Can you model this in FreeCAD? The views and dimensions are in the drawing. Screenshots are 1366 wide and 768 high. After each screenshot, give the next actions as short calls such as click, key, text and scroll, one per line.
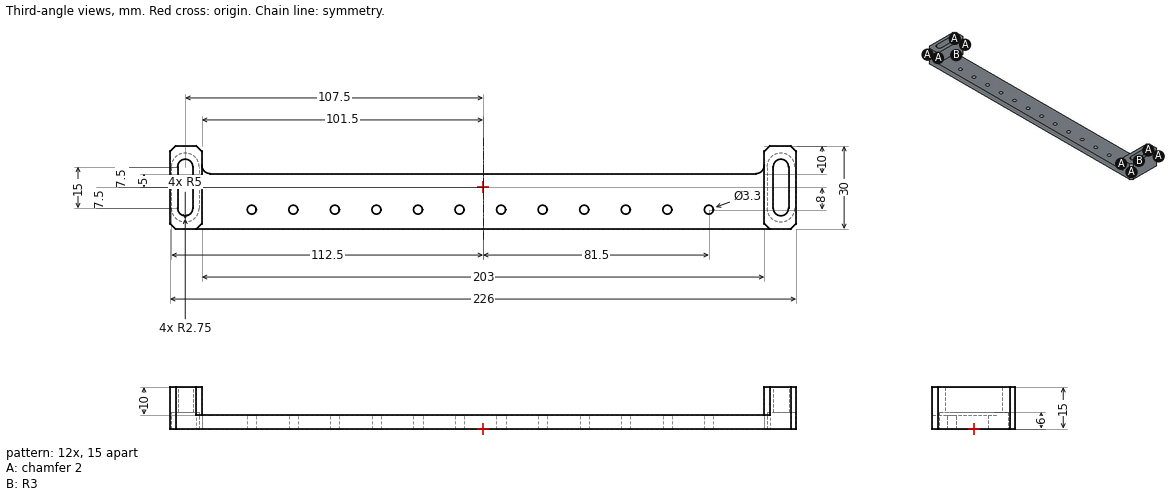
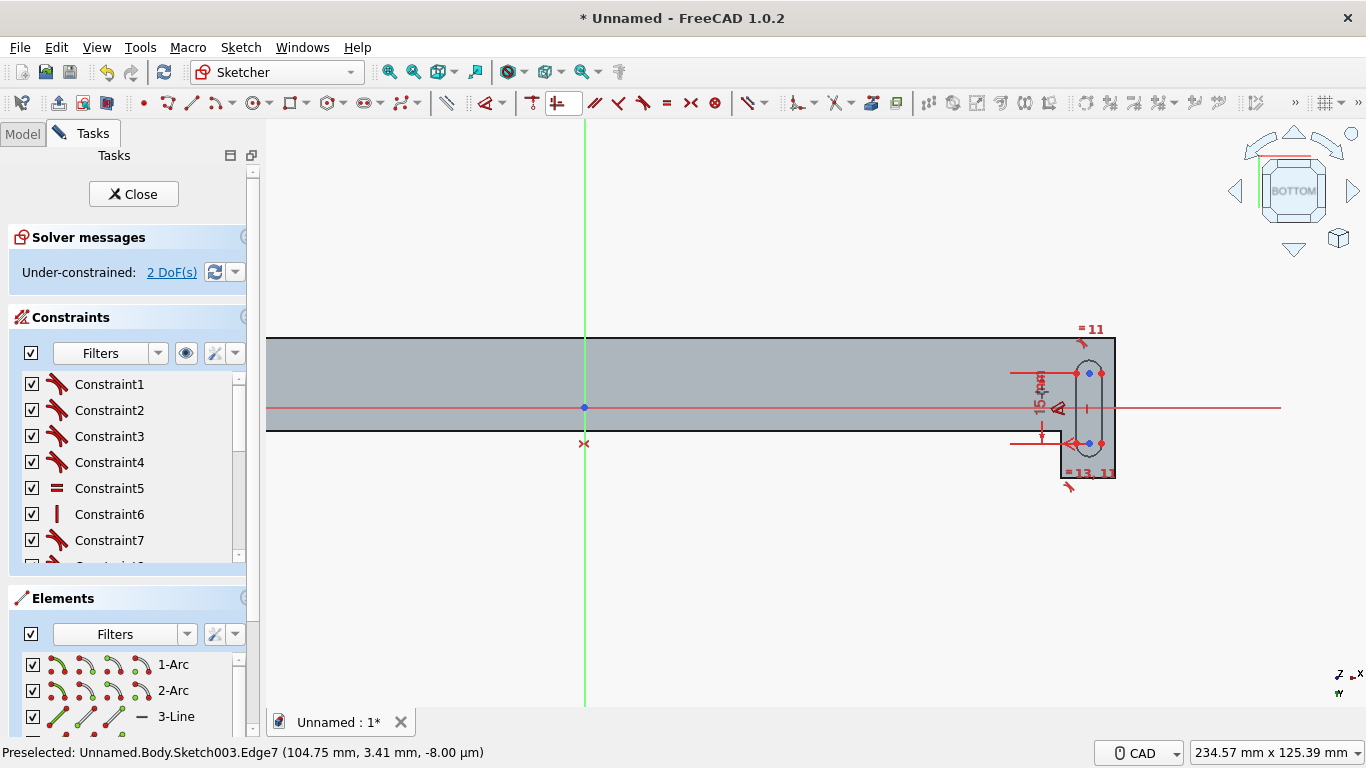
scroll(1078, 423, down, 2)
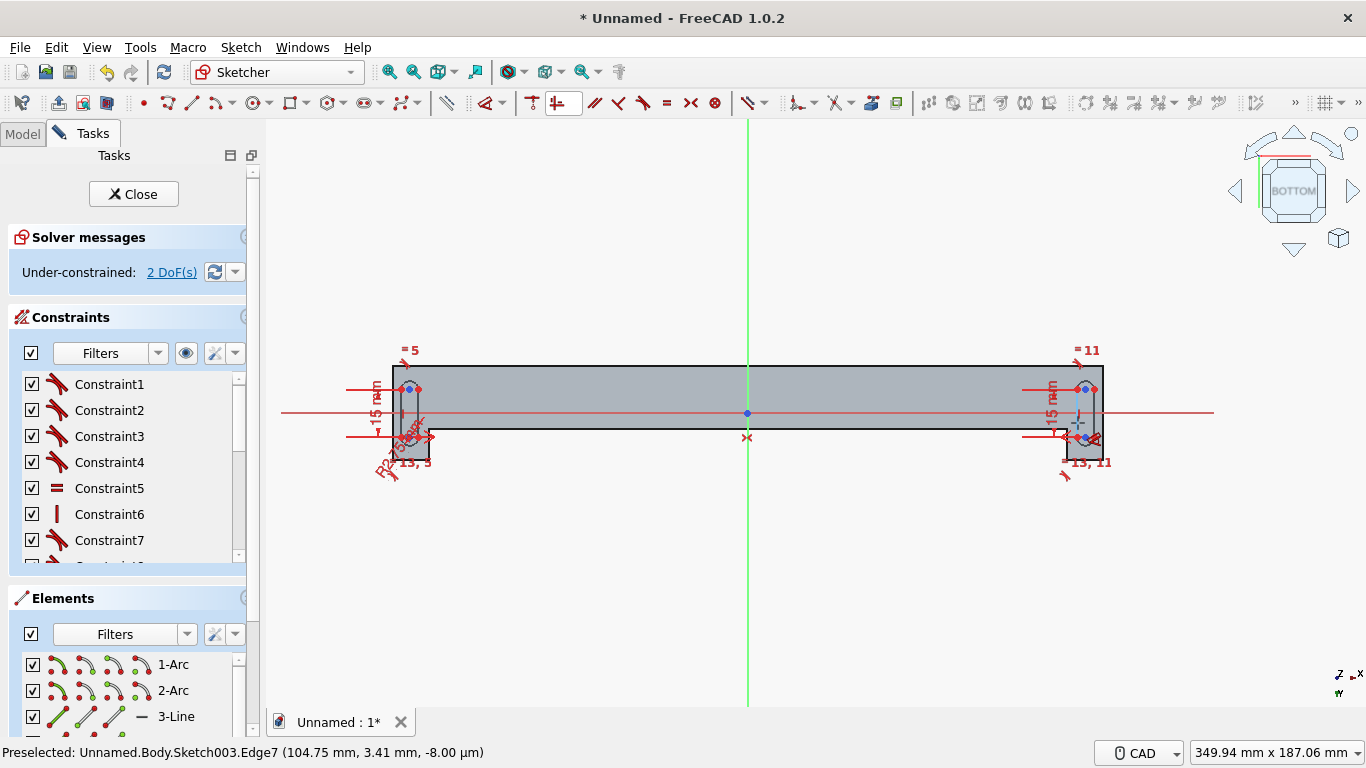
scroll(401, 437, up, 3)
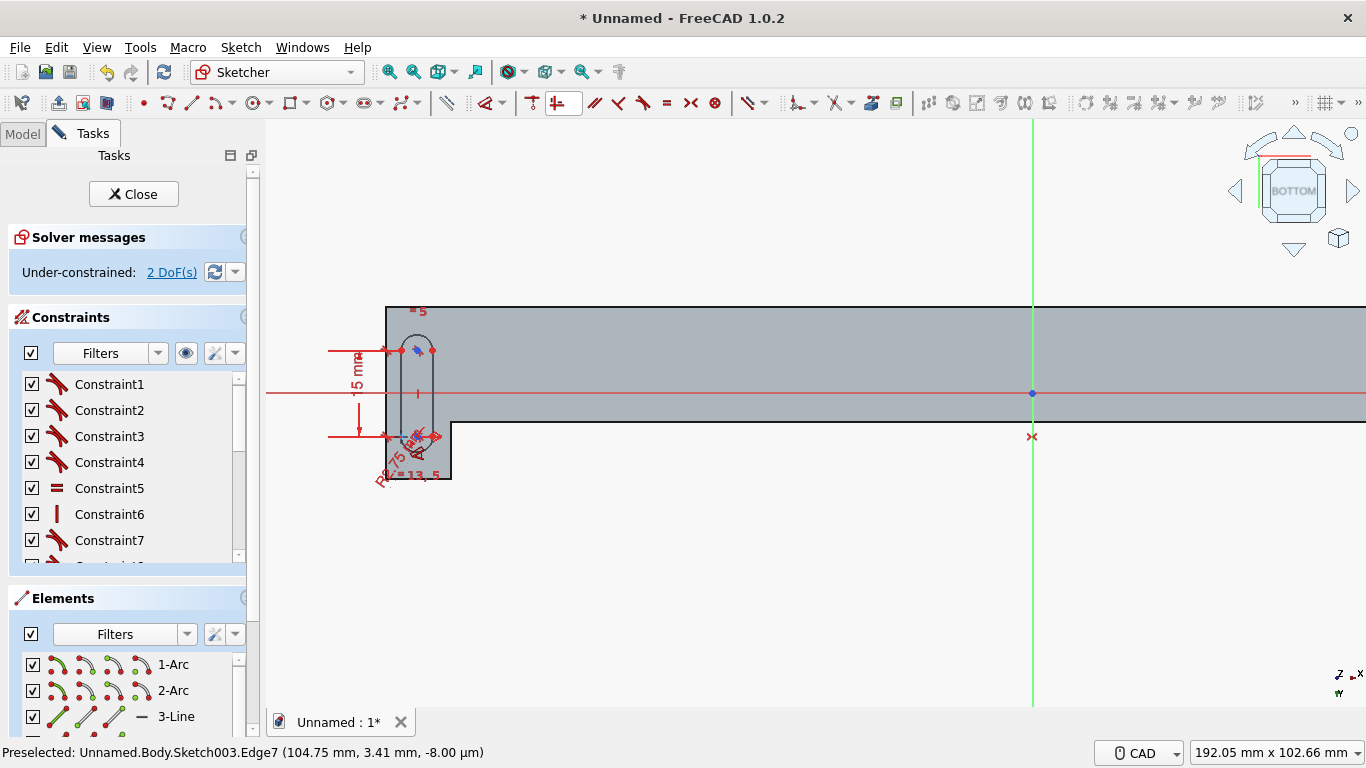
click(401, 437)
click(367, 415)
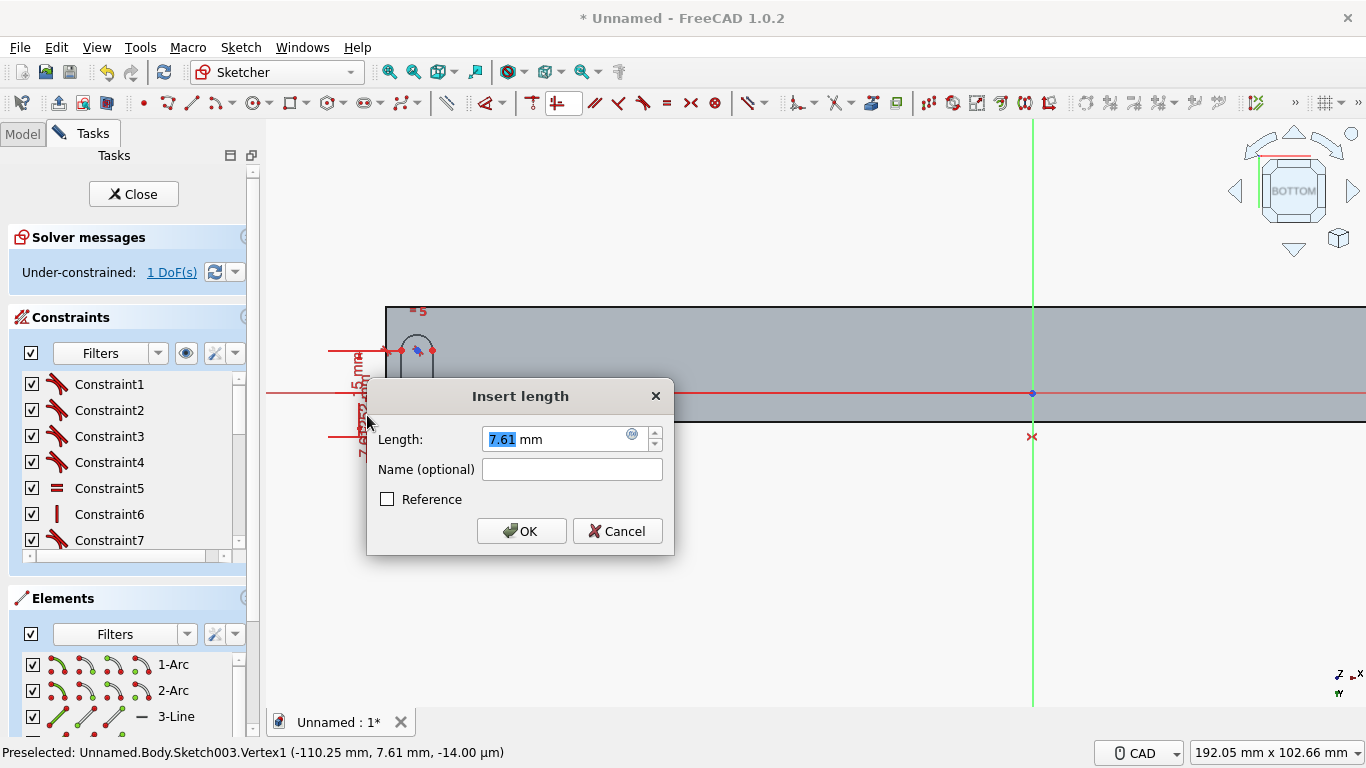
text(7.5)
key(Return)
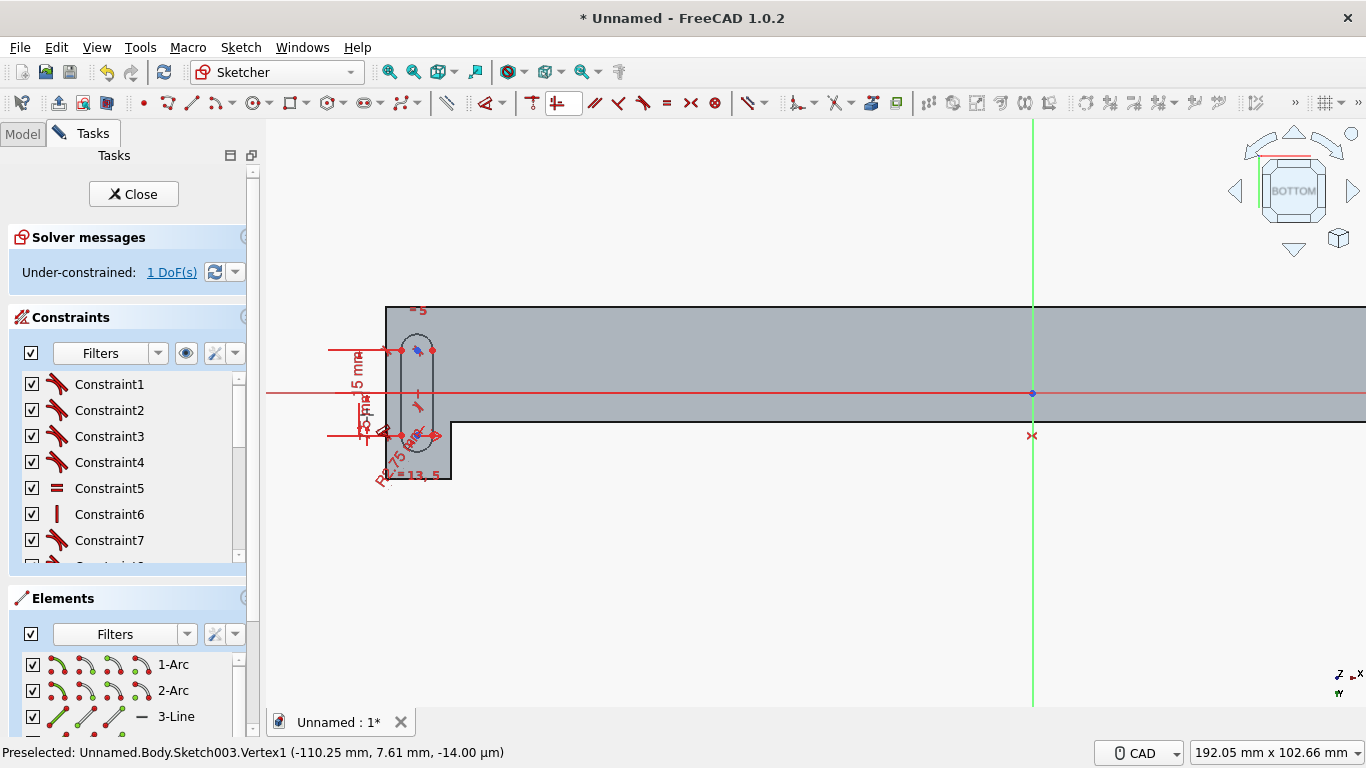
click(417, 436)
click(725, 470)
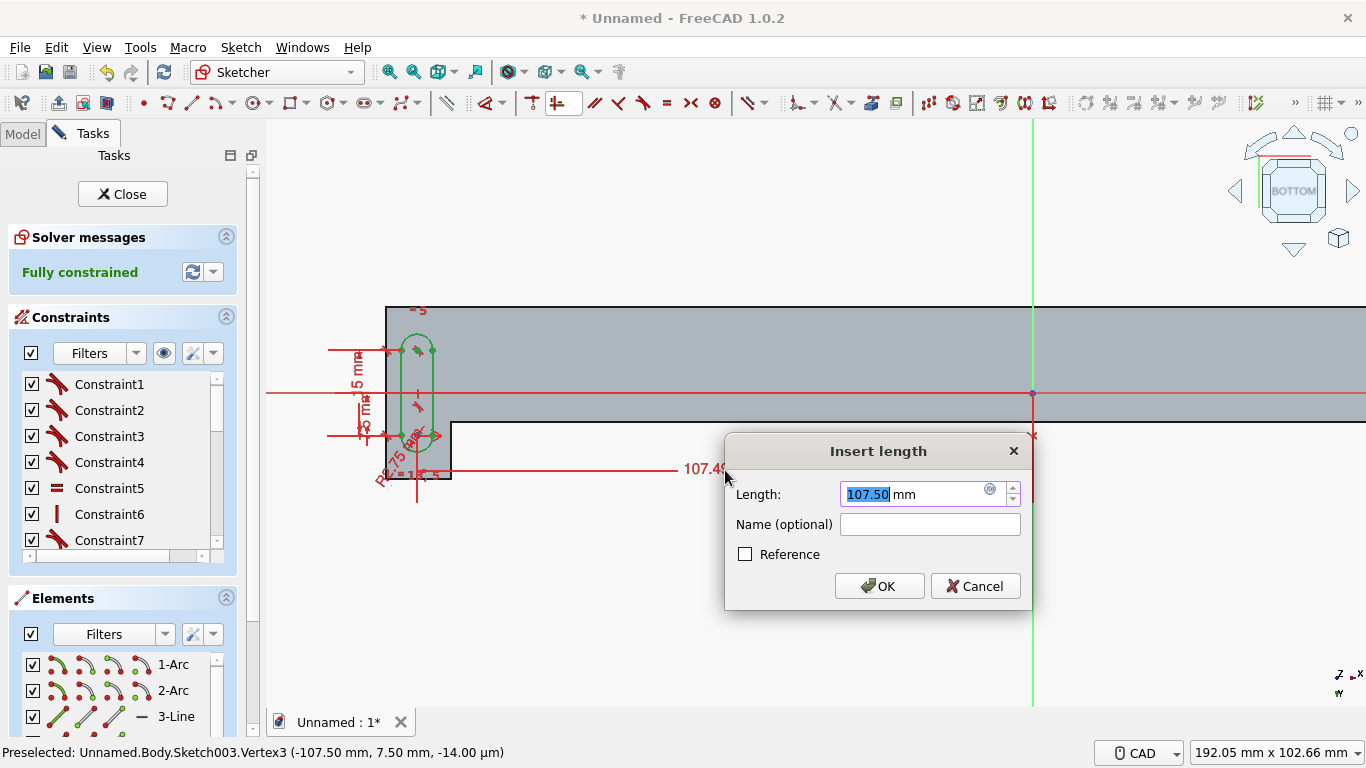
text(107.5)
key(Return)
key(Escape)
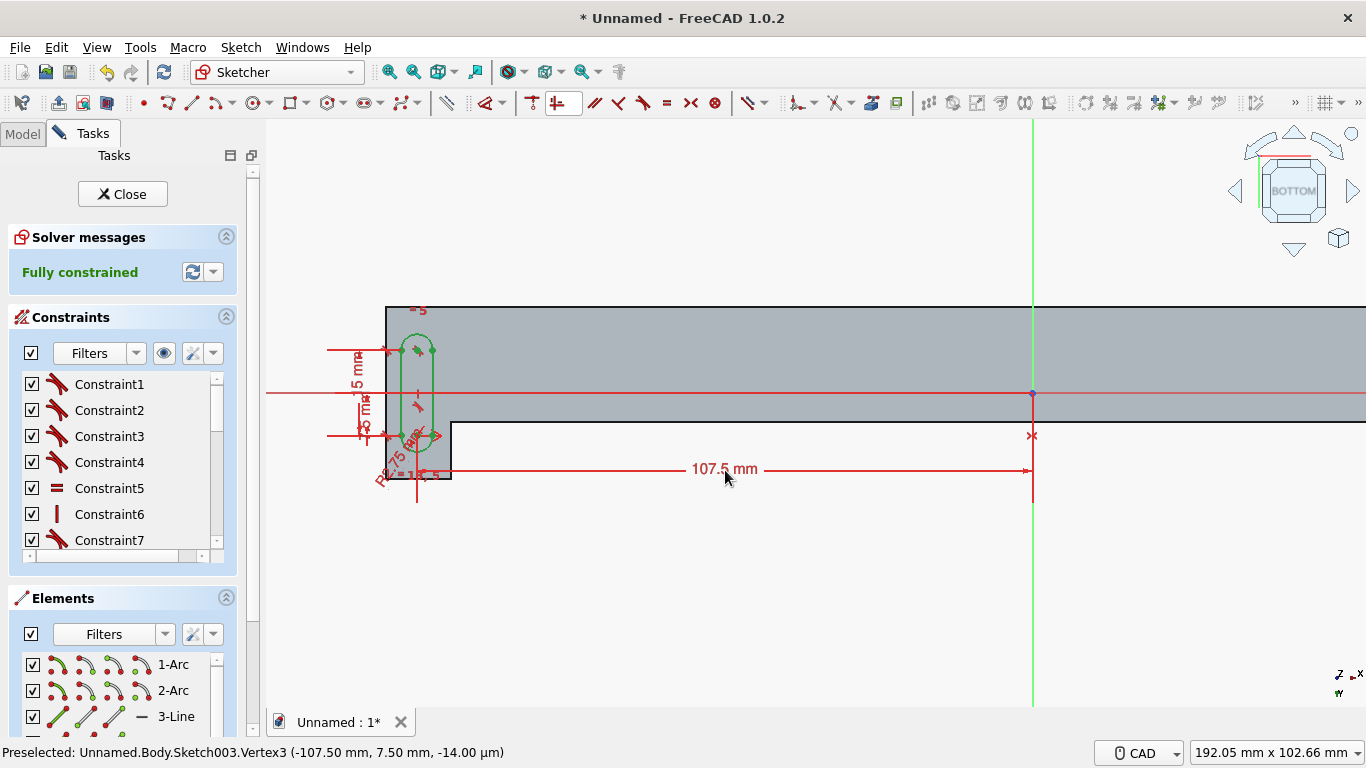
click(123, 194)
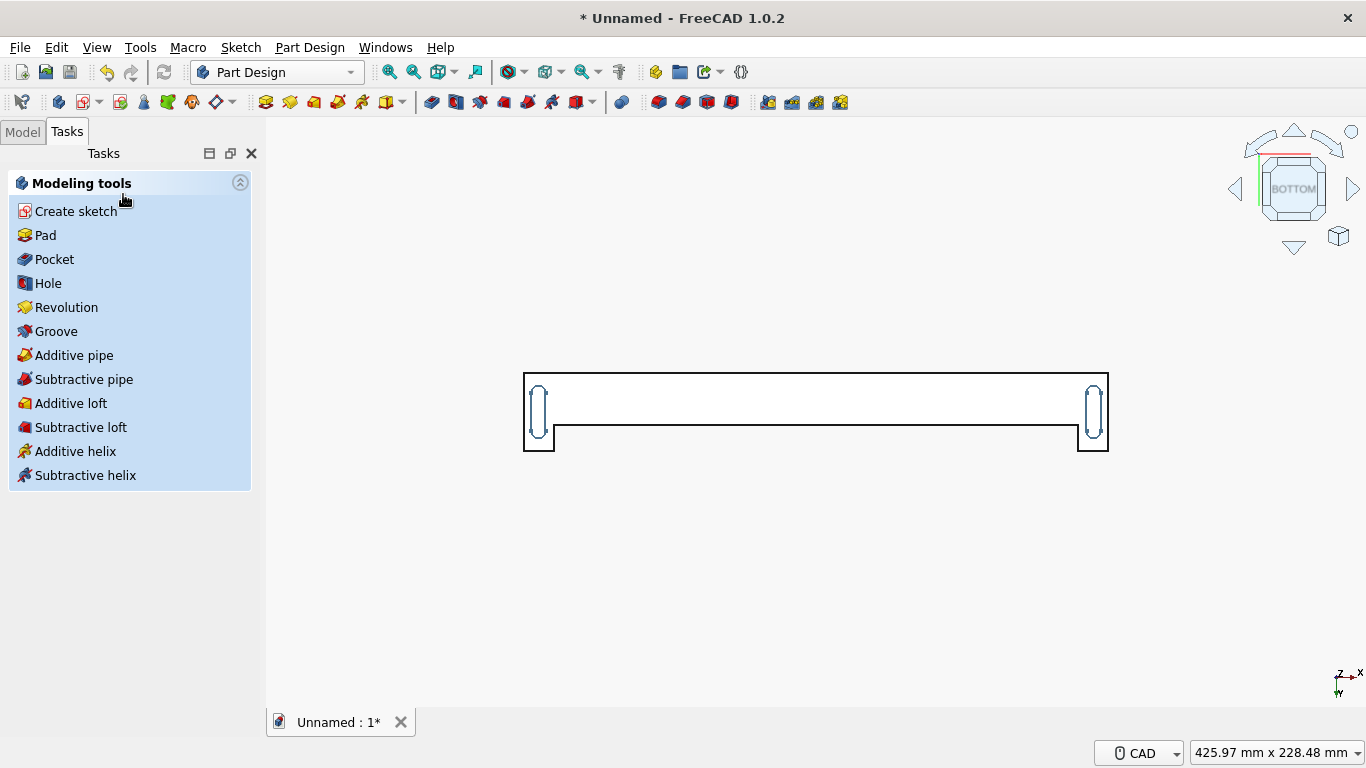
click(432, 102)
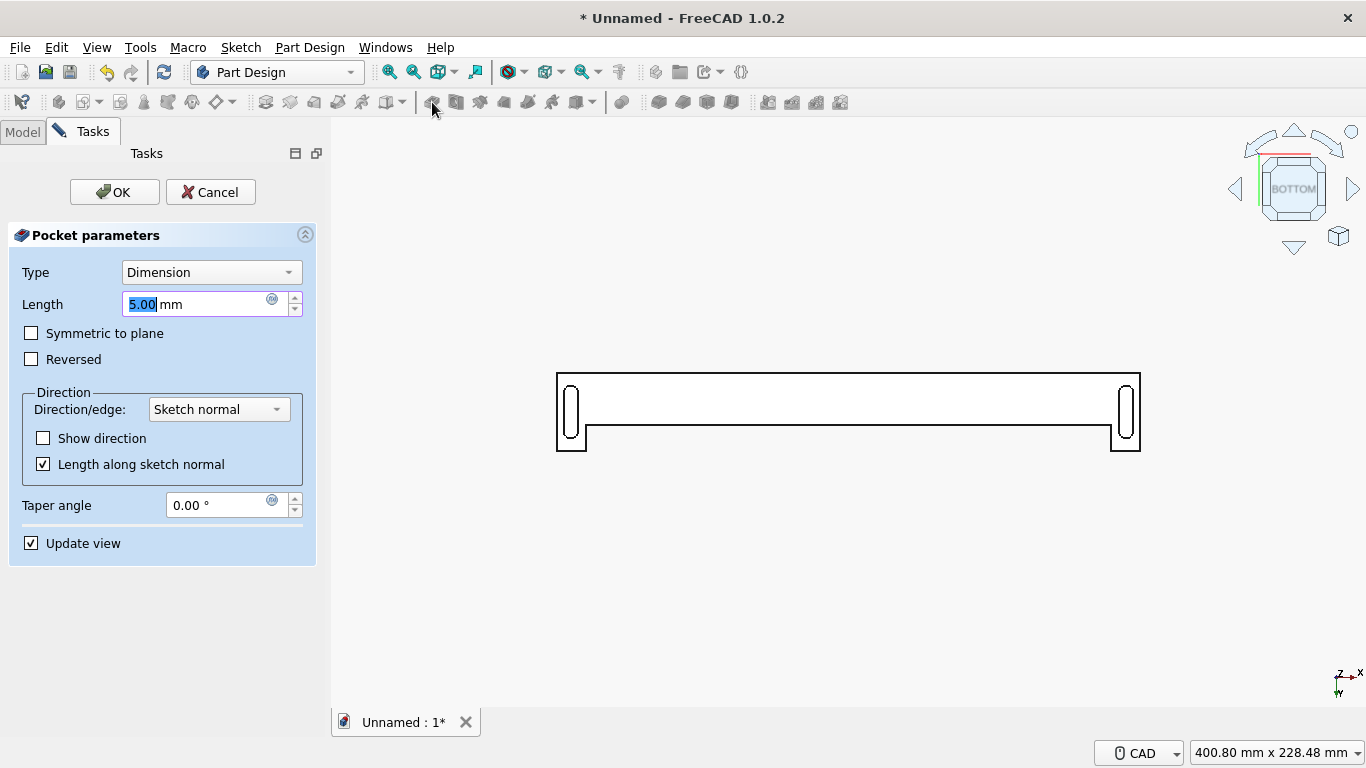
click(212, 272)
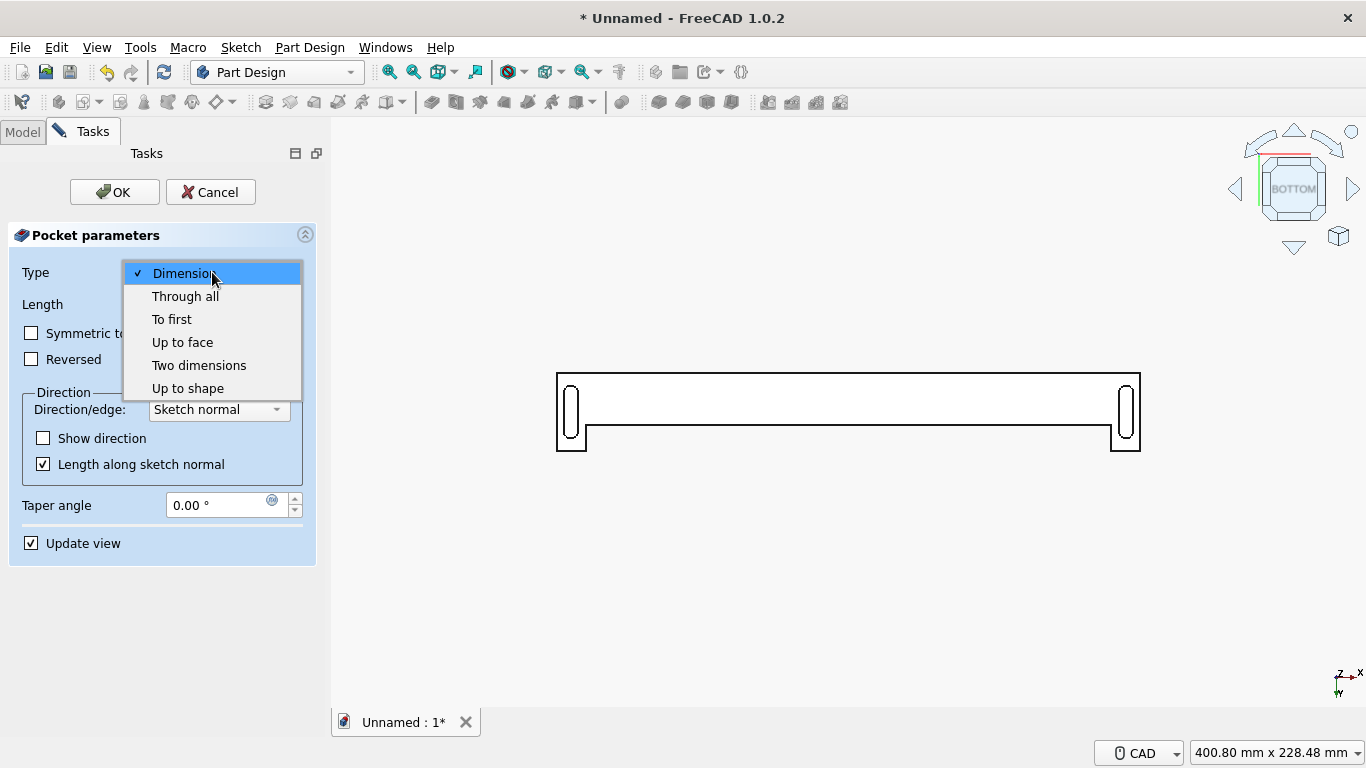
click(212, 296)